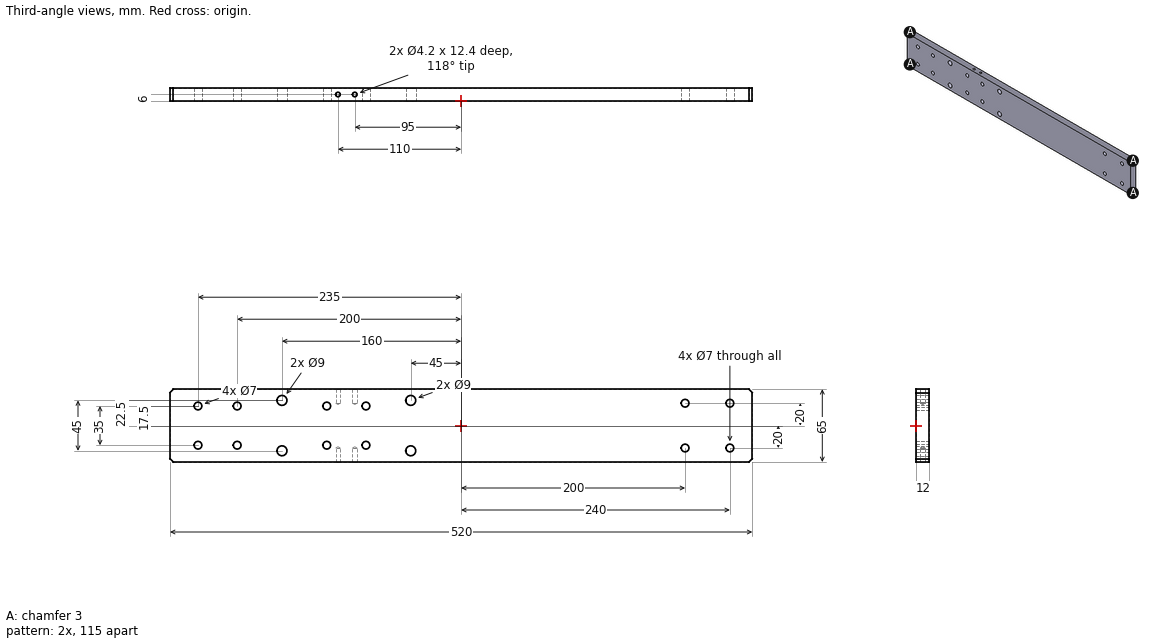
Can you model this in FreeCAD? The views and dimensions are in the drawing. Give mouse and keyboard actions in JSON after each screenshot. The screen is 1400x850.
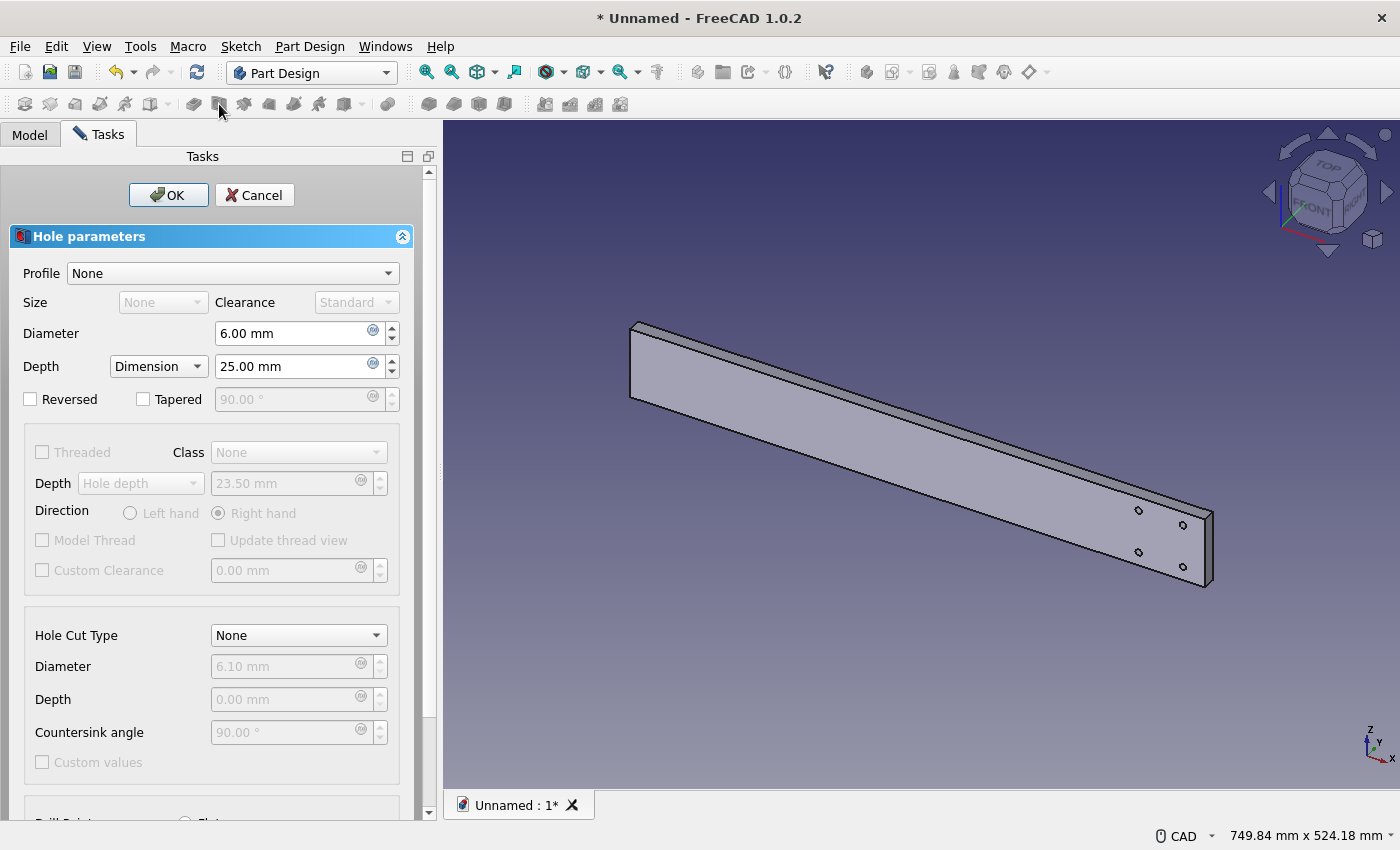
{"action": "triple_click", "coordinate": [300, 334]}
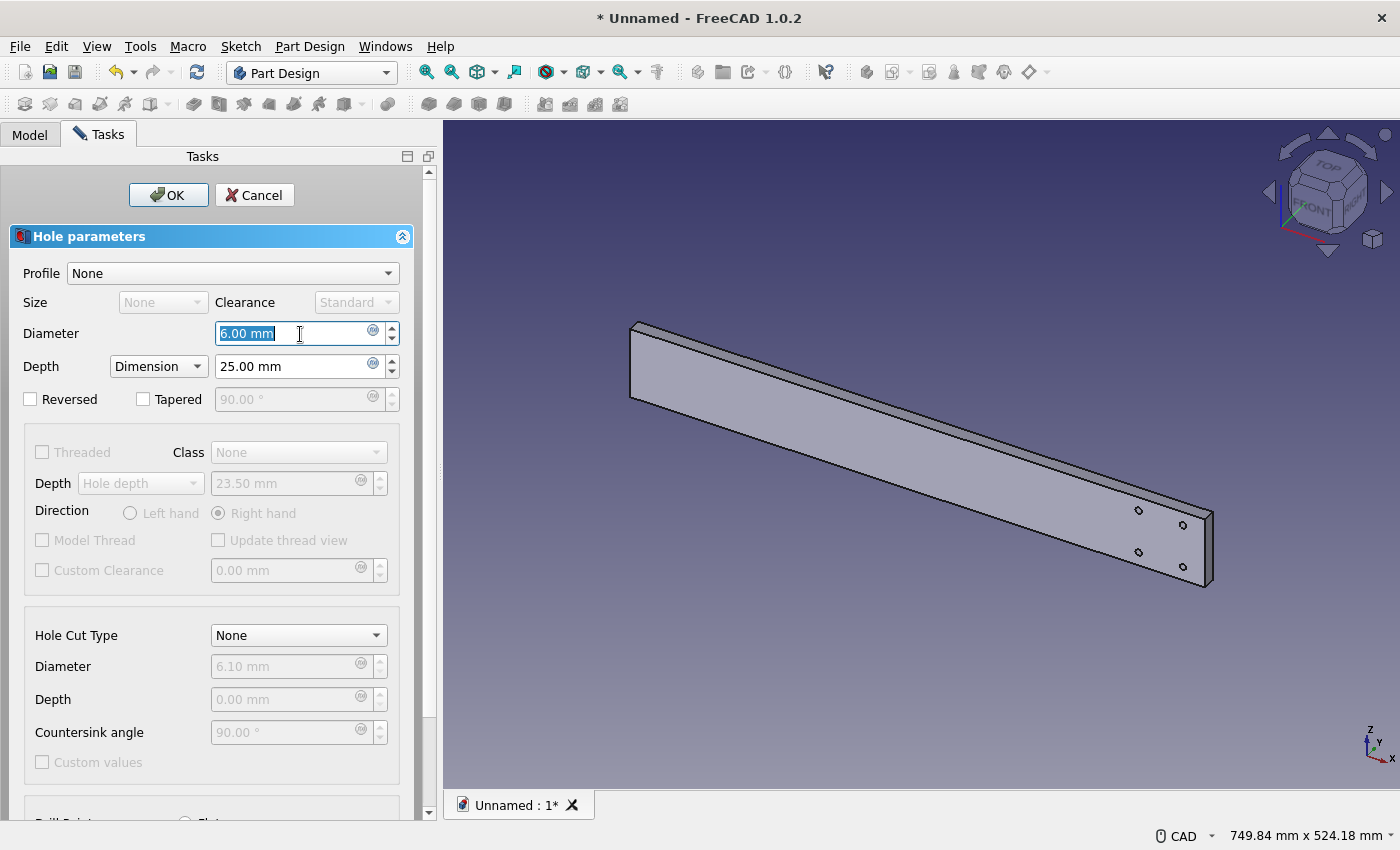
{"action": "type", "text": "7"}
{"action": "key", "text": "Tab"}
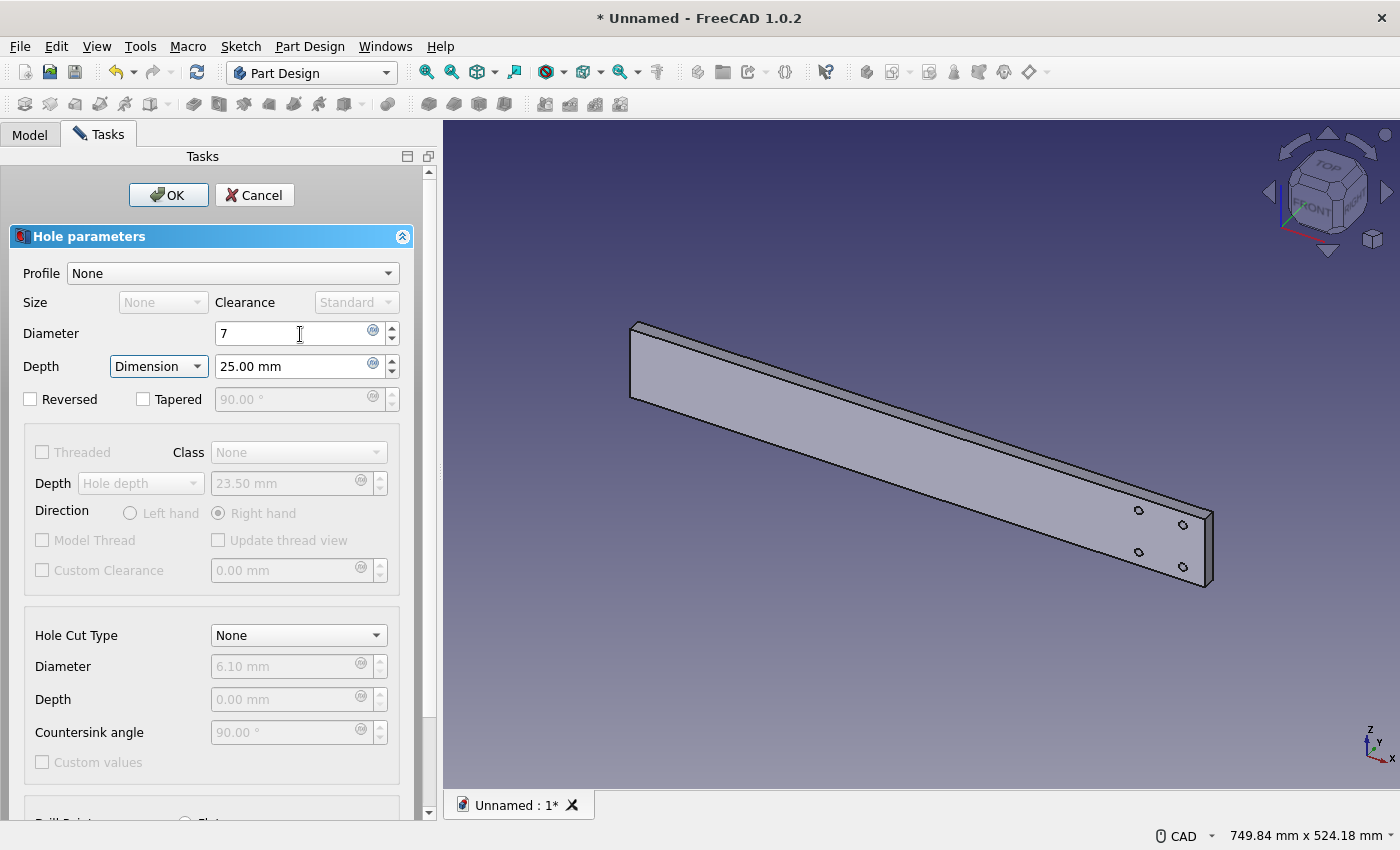
{"action": "left_click", "coordinate": [160, 366]}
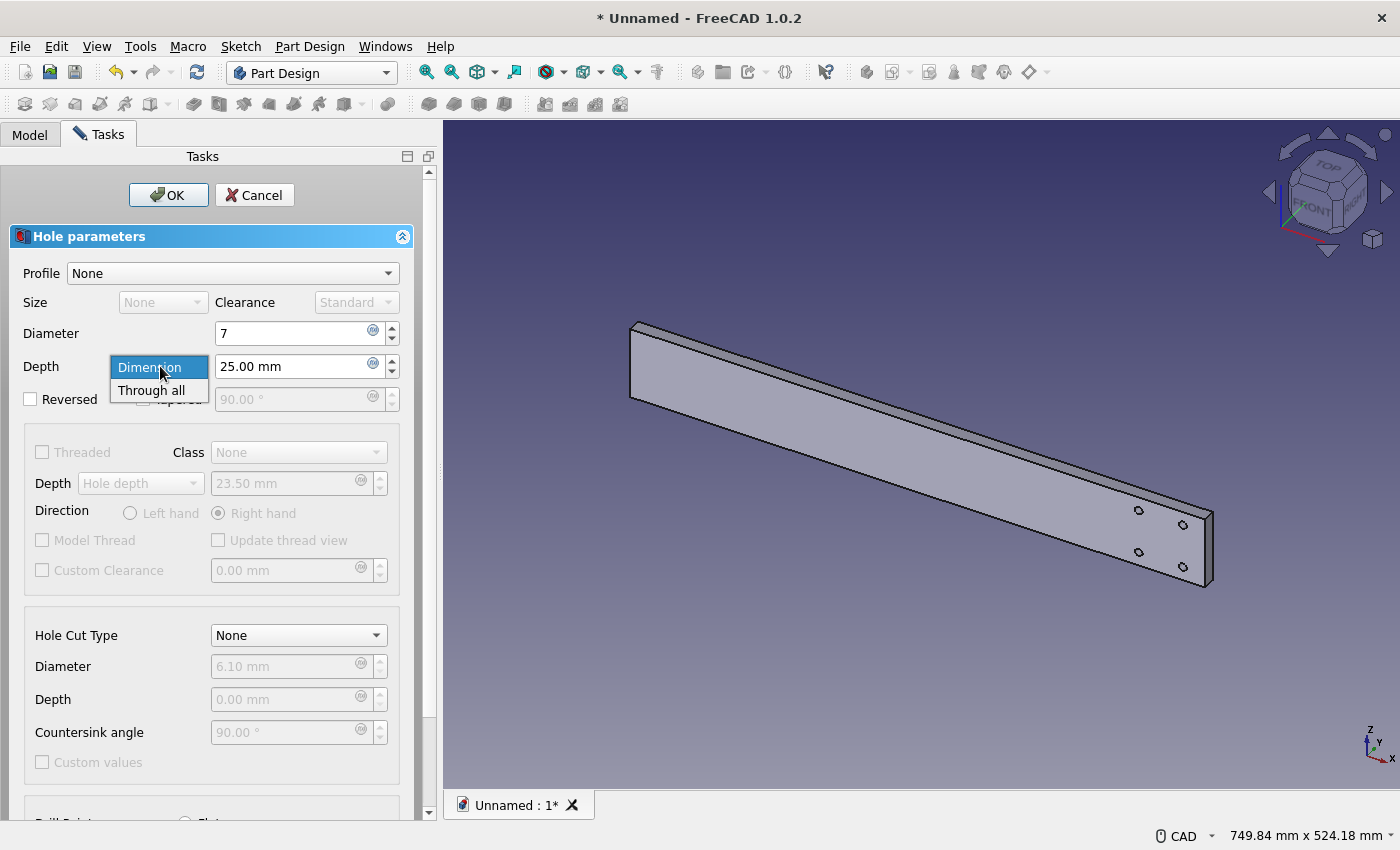
{"action": "left_click", "coordinate": [158, 390]}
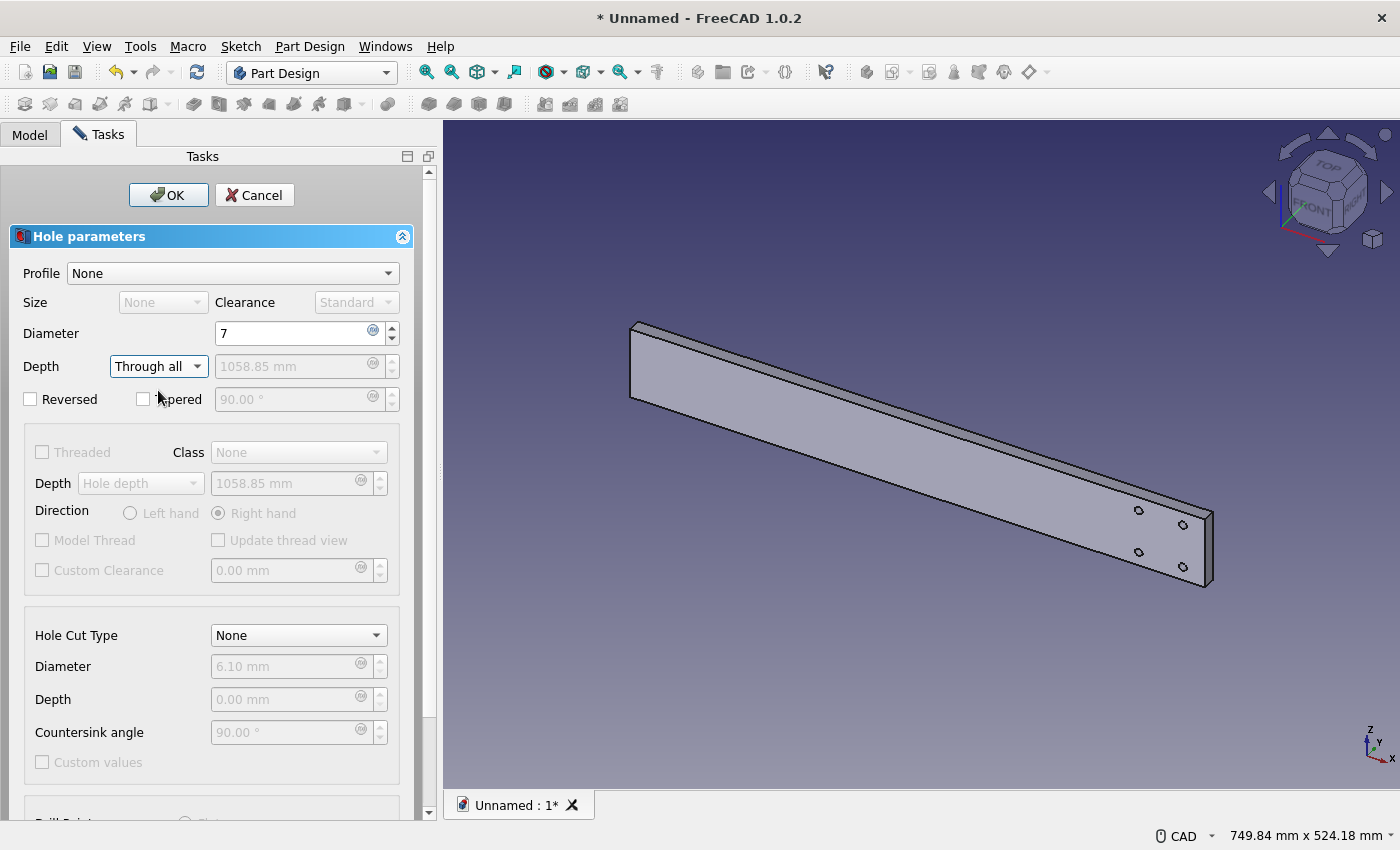
{"action": "left_click", "coordinate": [169, 195]}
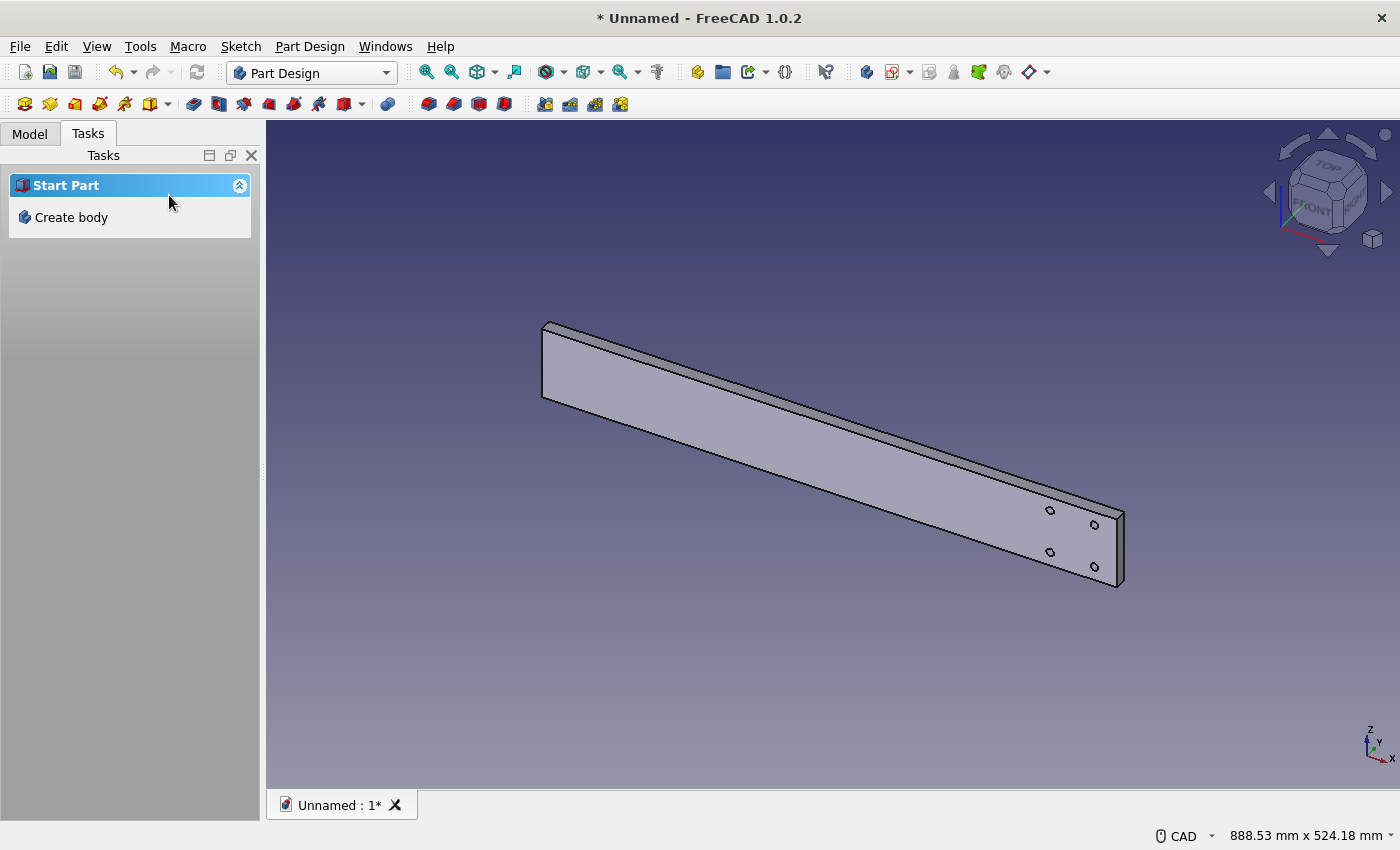
{"action": "left_click", "coordinate": [1122, 513]}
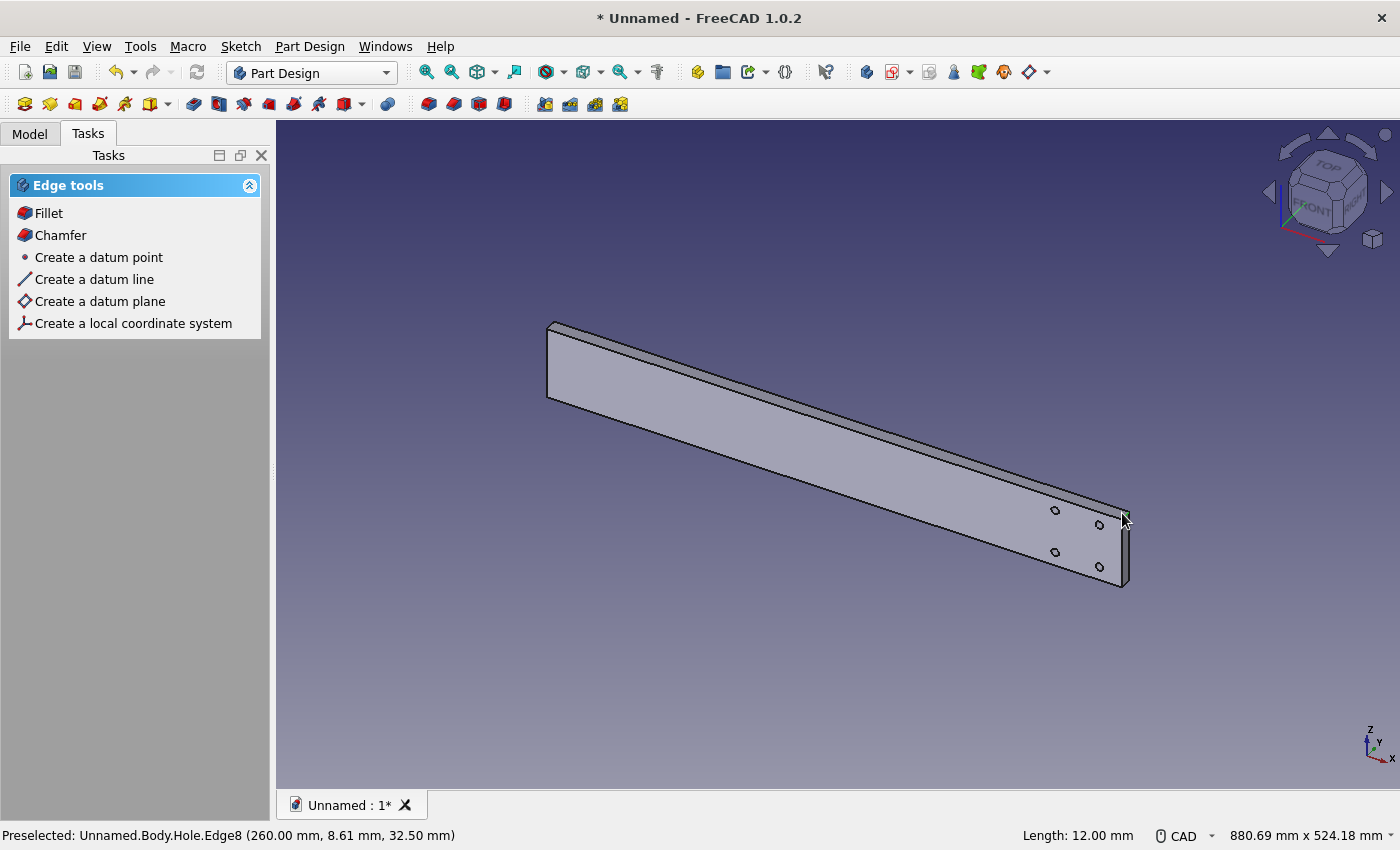
{"action": "scroll", "coordinate": [551, 324], "scroll_direction": "up", "scroll_amount": 5}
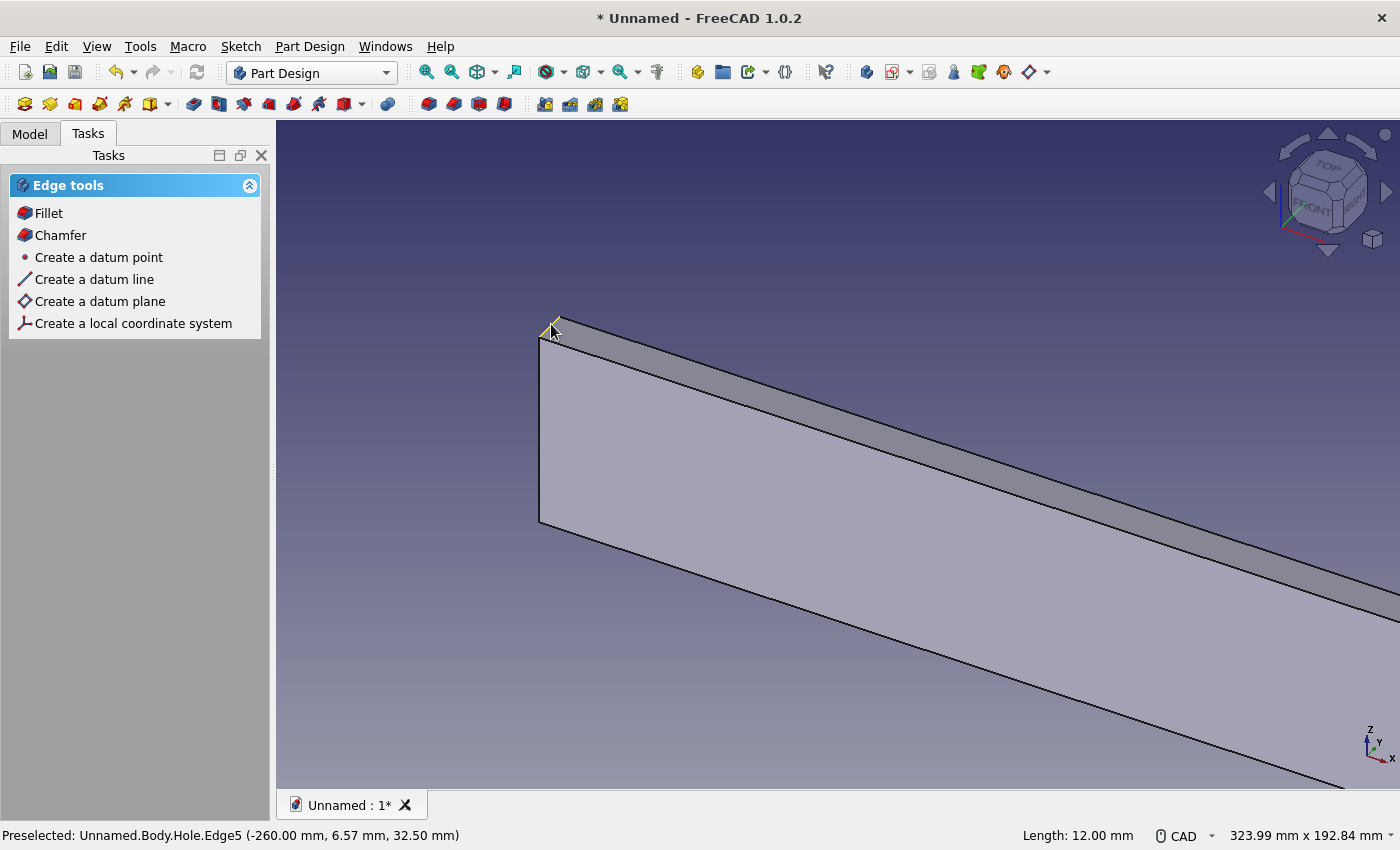
{"action": "key", "text": "v f"}